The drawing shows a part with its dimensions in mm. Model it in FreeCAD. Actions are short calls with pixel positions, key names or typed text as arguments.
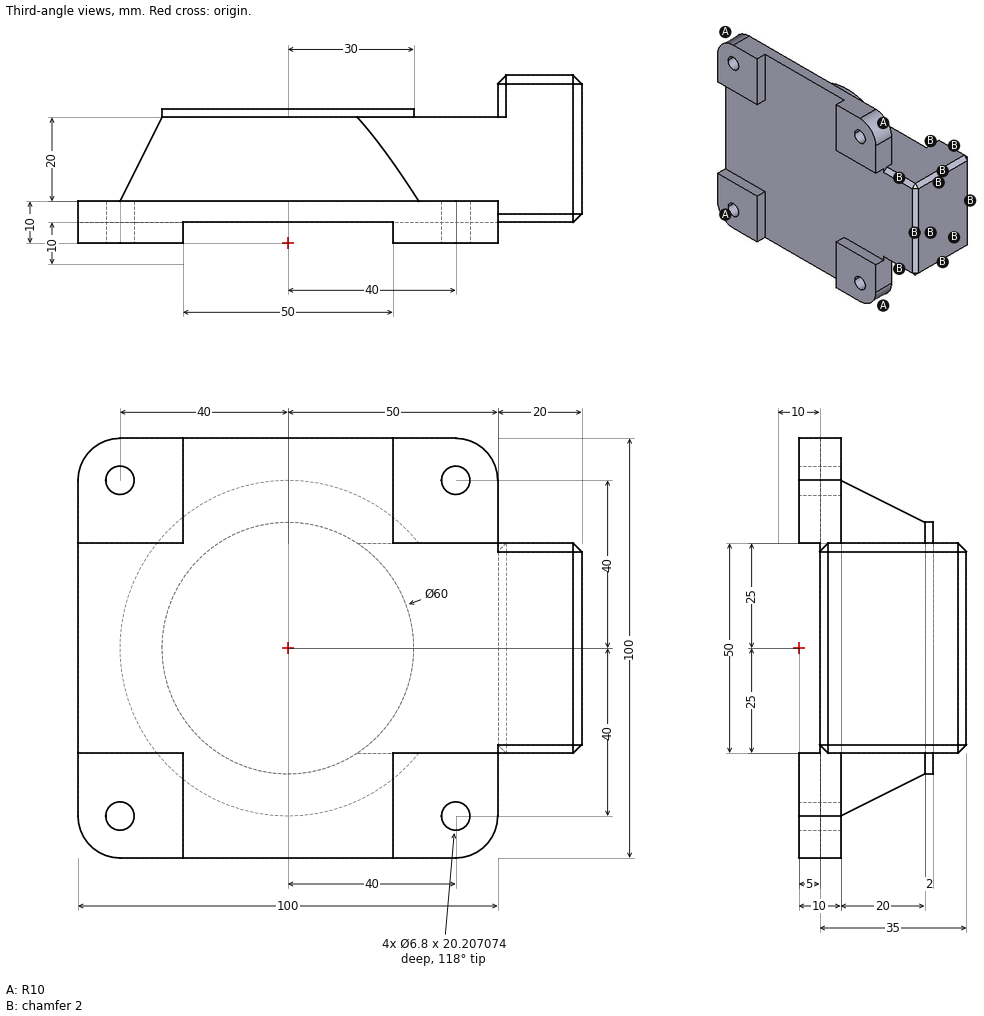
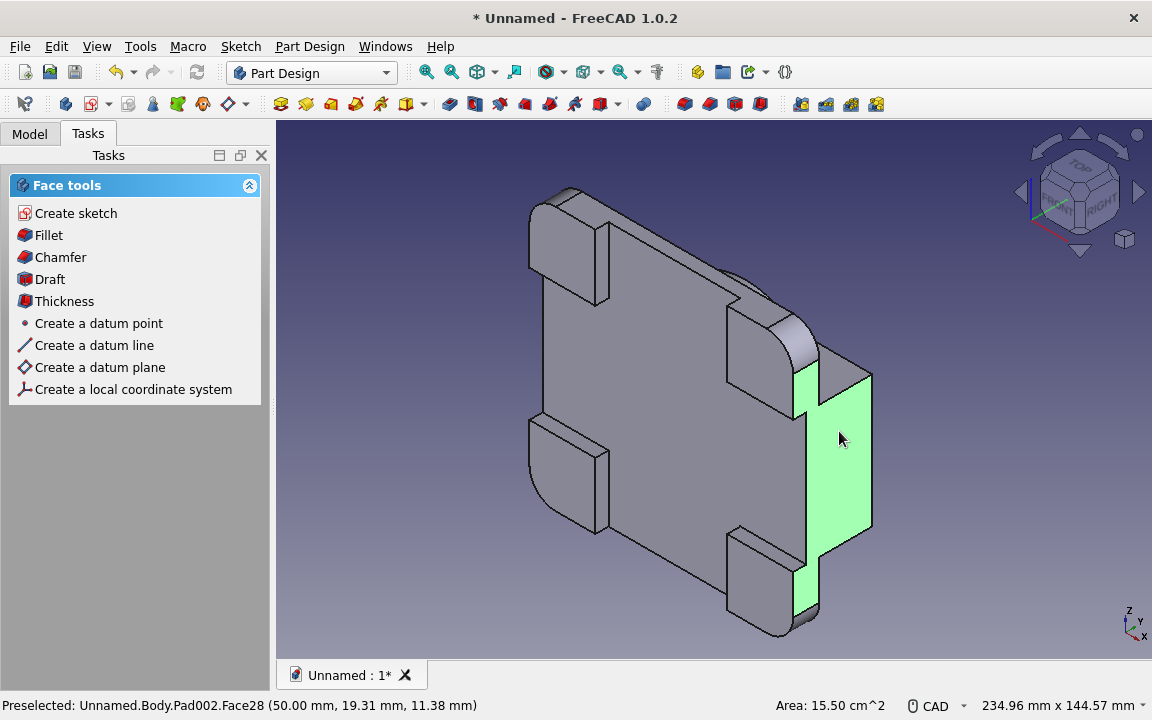
click(90, 104)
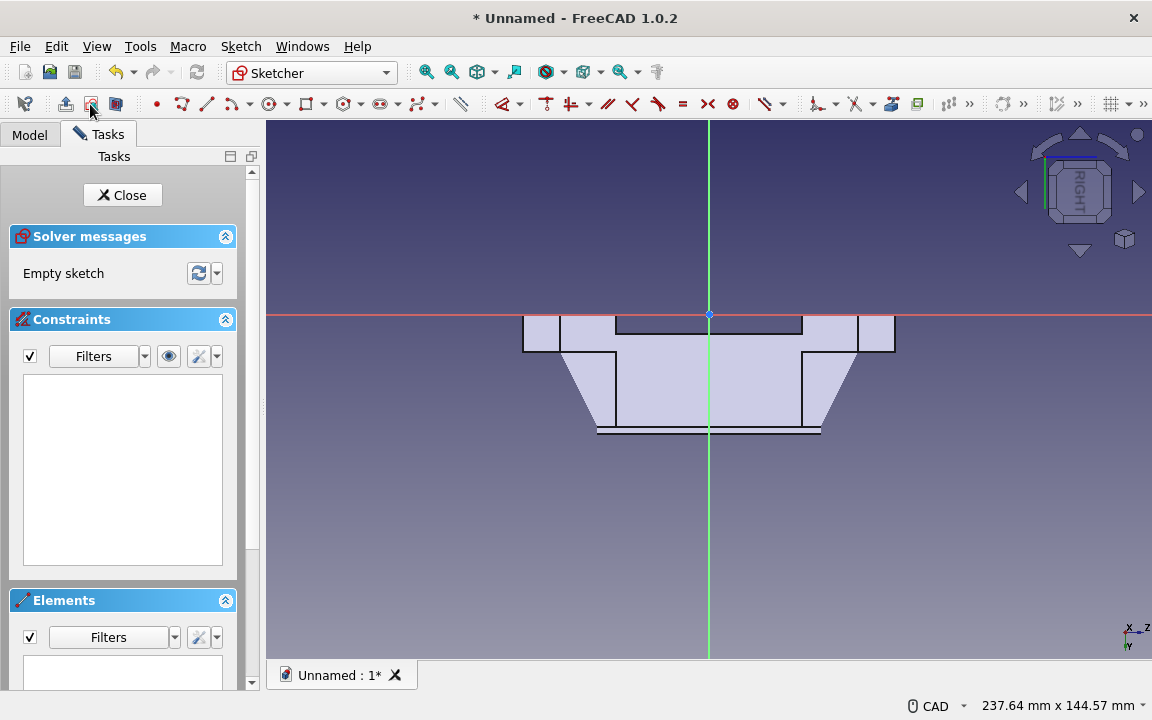
scroll(765, 390, up, 4)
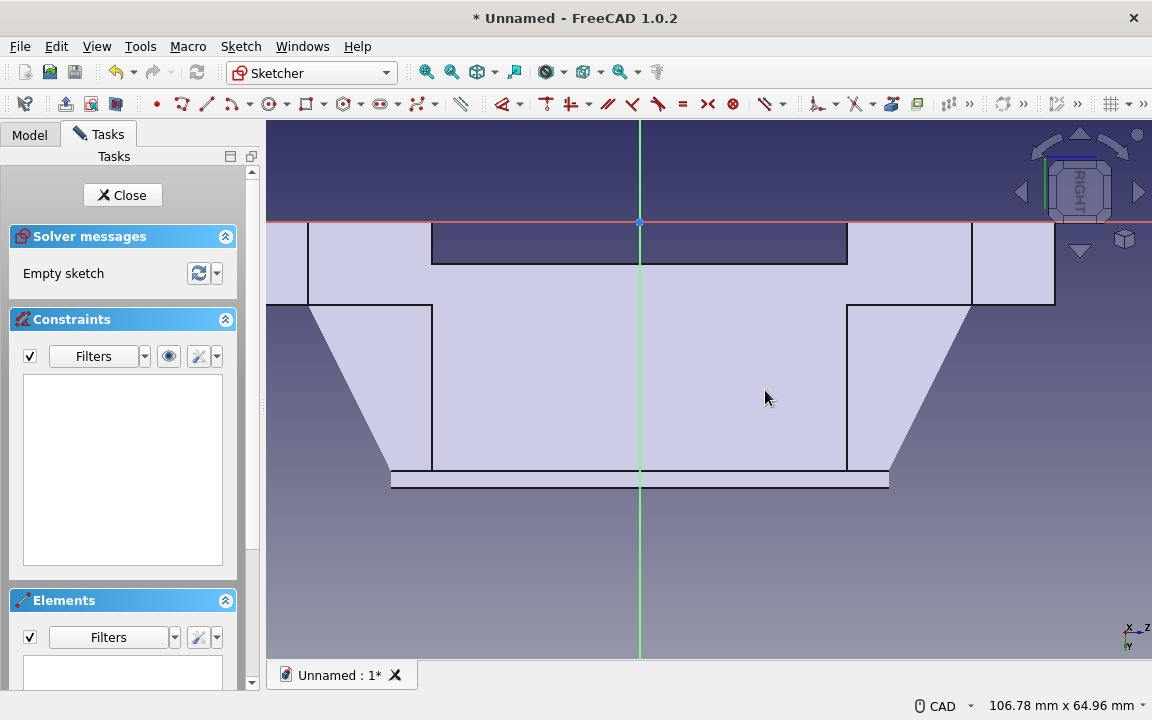
click(306, 104)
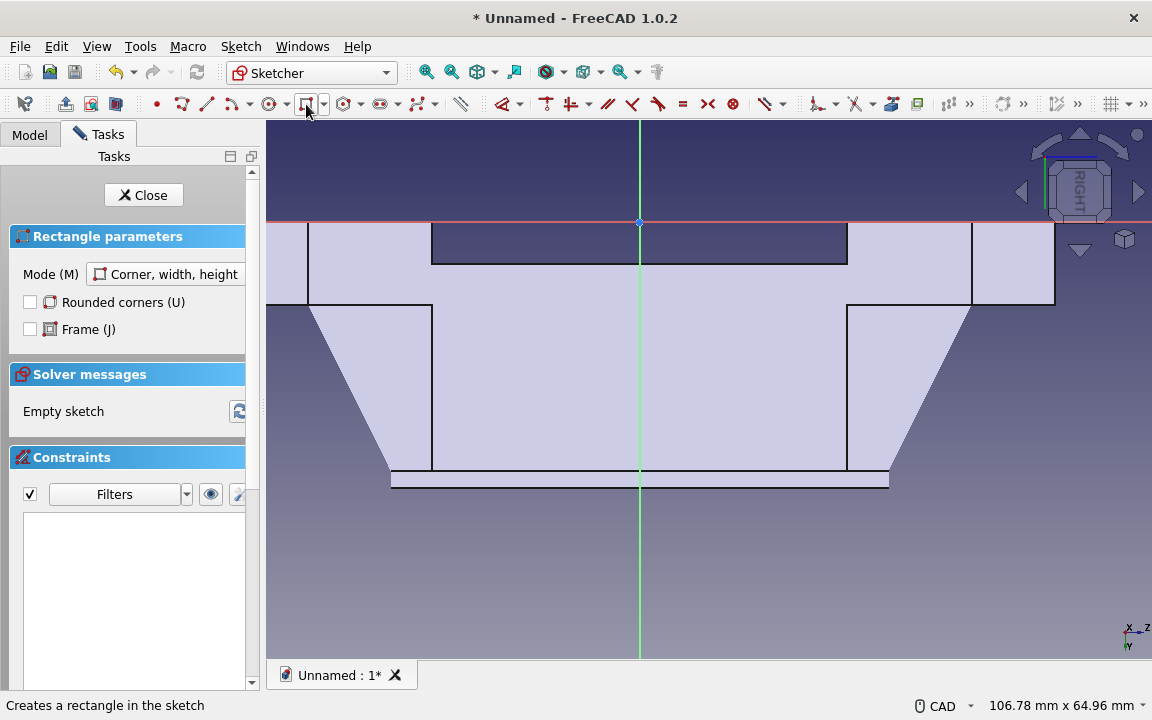
click(432, 264)
click(847, 554)
key(Escape)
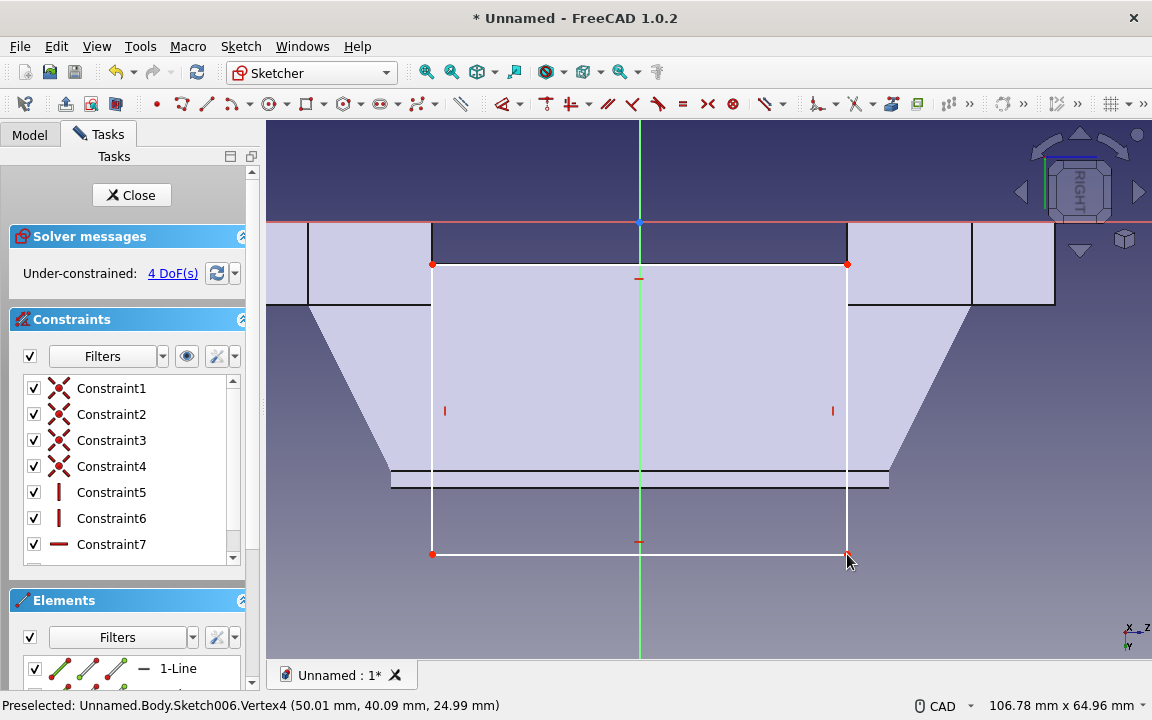
click(502, 104)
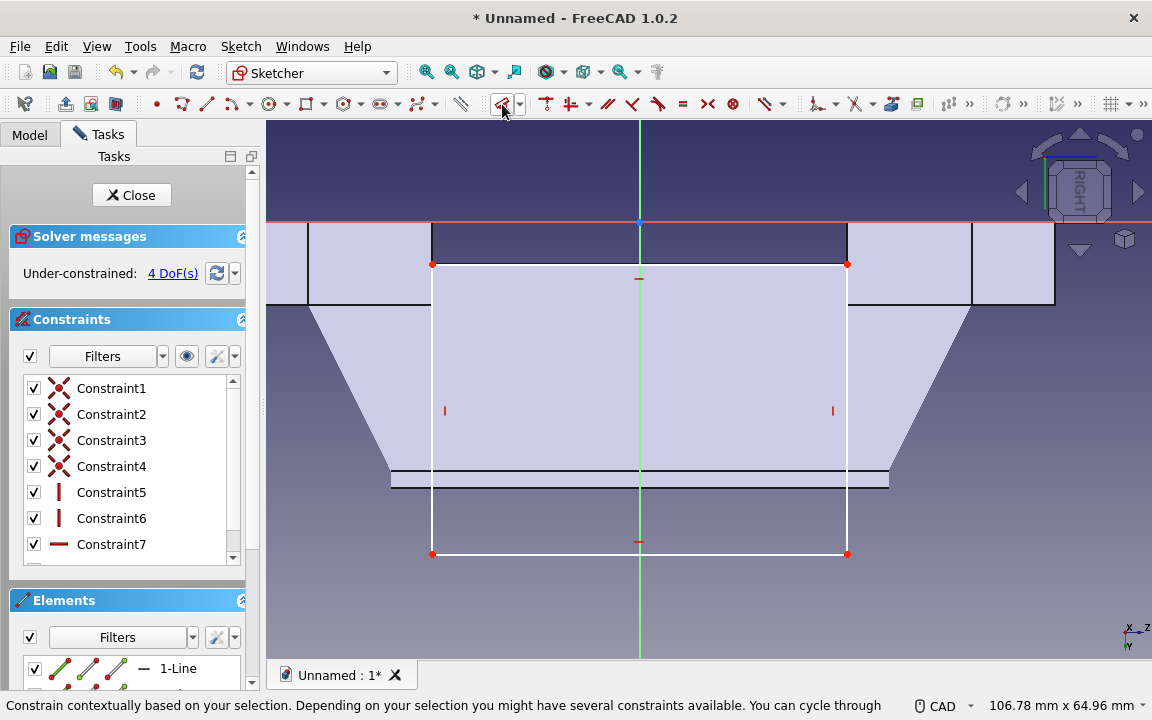
click(432, 352)
click(398, 410)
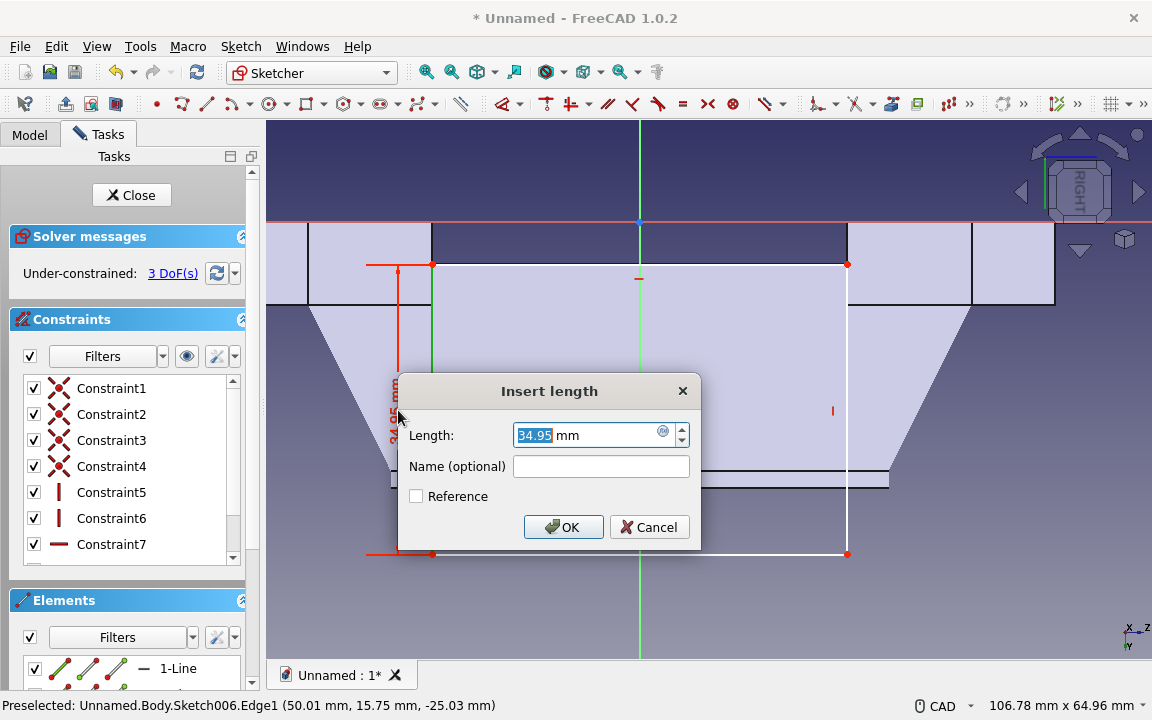
text(35)
key(Return)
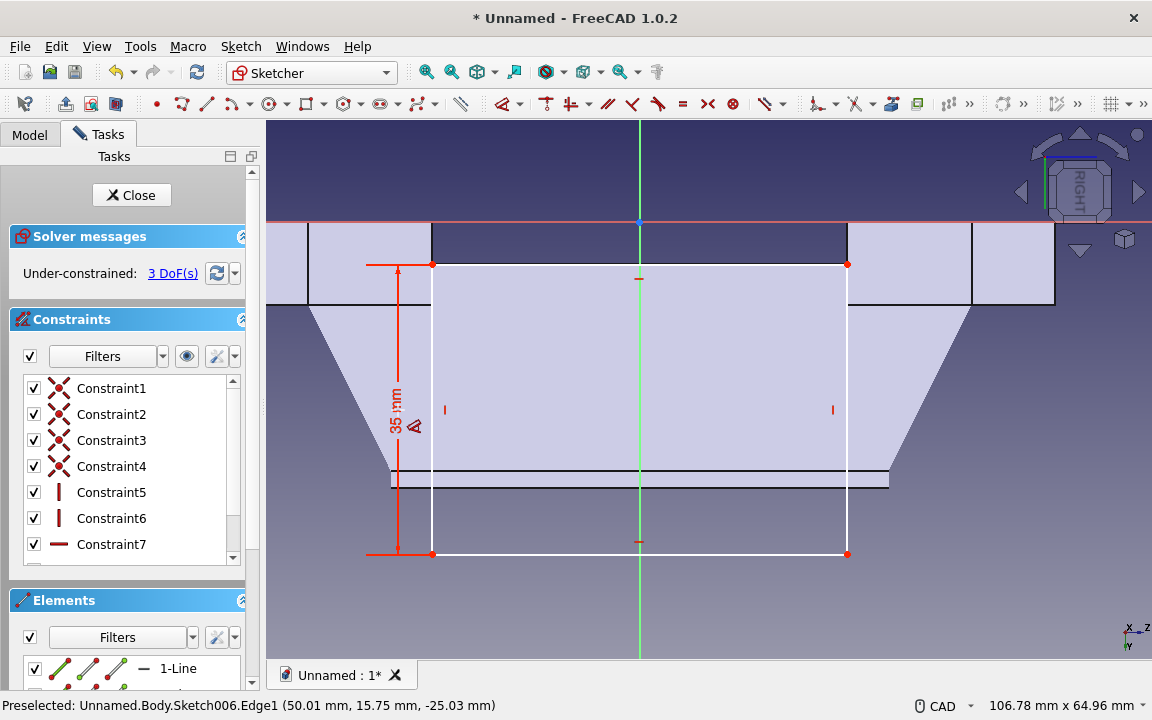
click(557, 555)
click(544, 589)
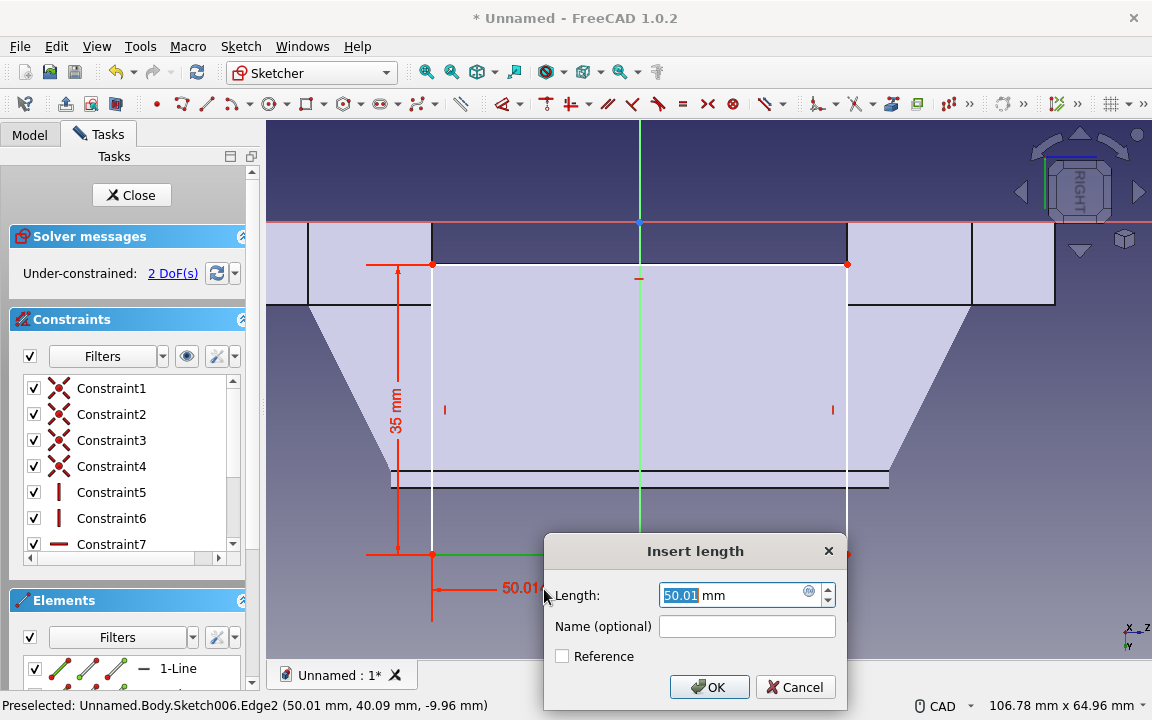
text(50)
key(Return)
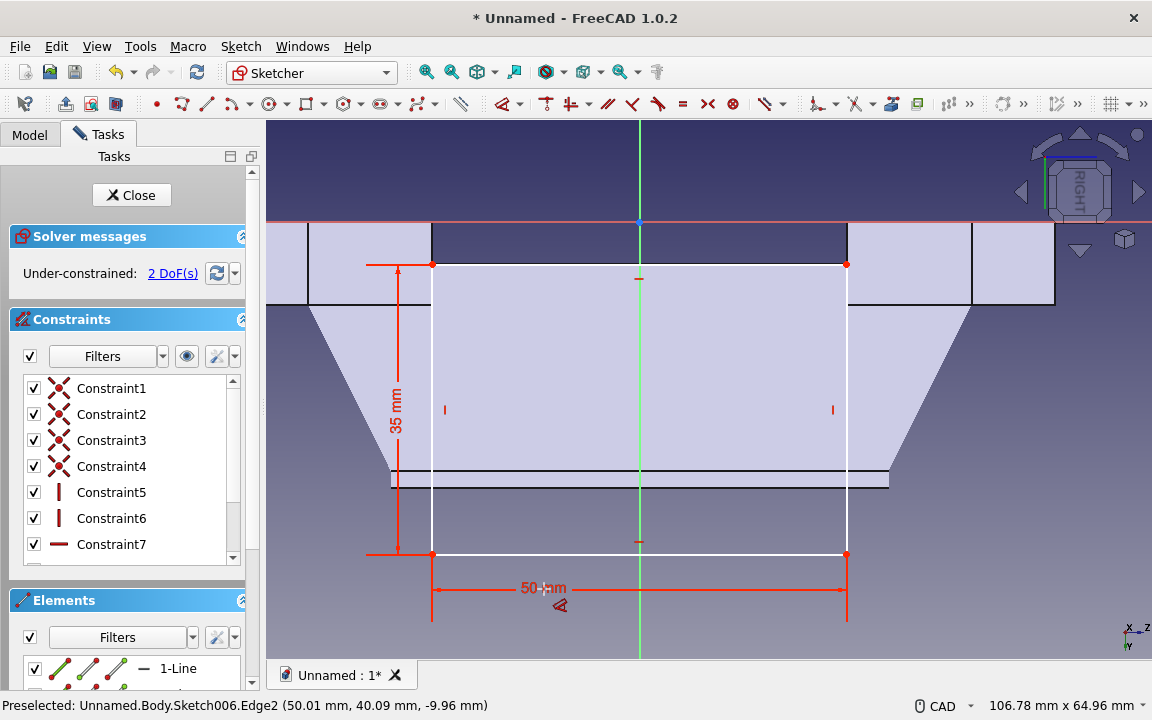
click(432, 265)
click(398, 243)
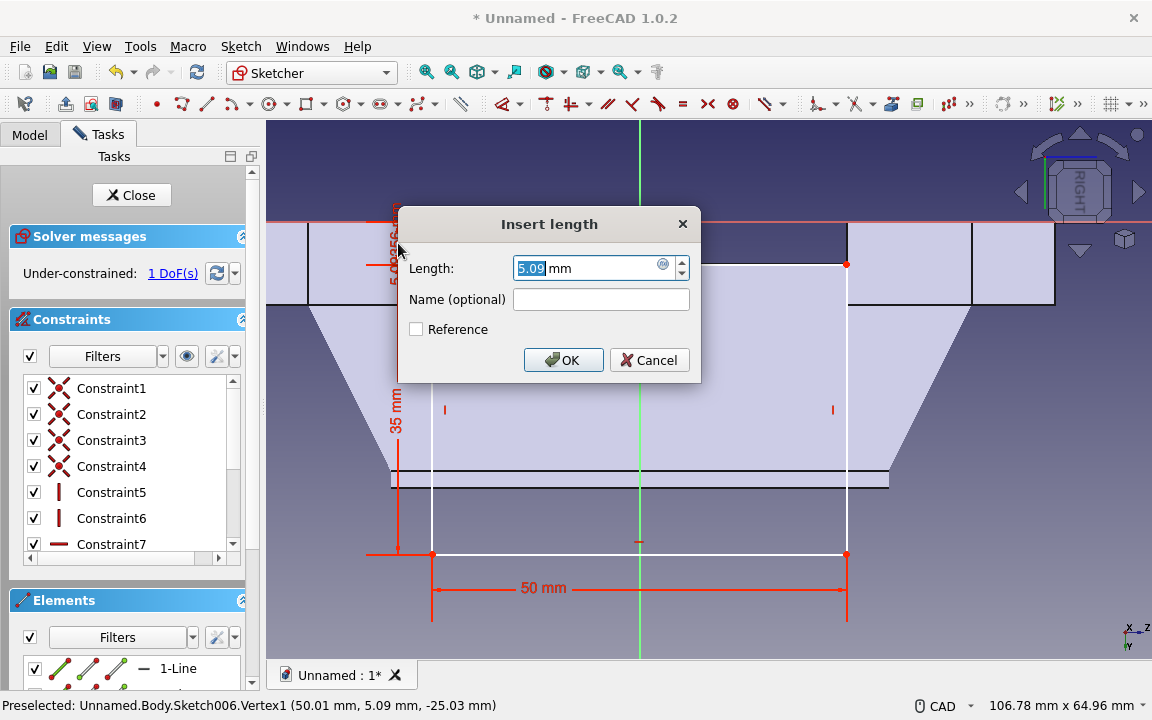
text(5)
key(Return)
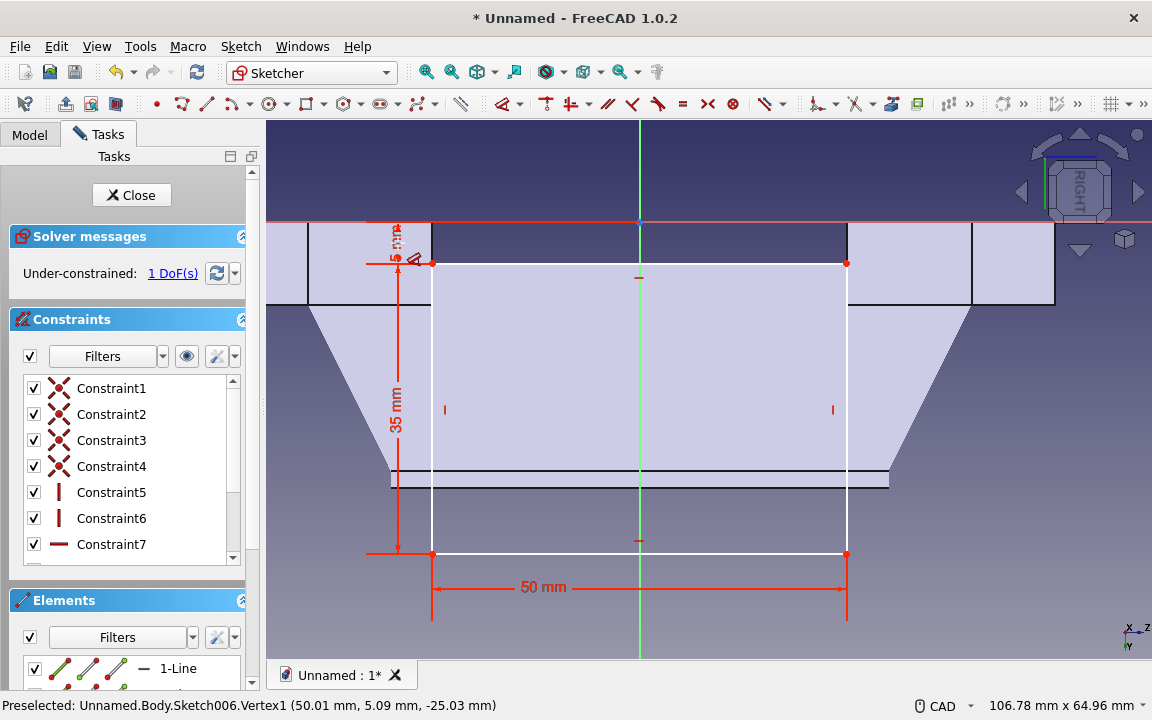
click(432, 264)
click(536, 188)